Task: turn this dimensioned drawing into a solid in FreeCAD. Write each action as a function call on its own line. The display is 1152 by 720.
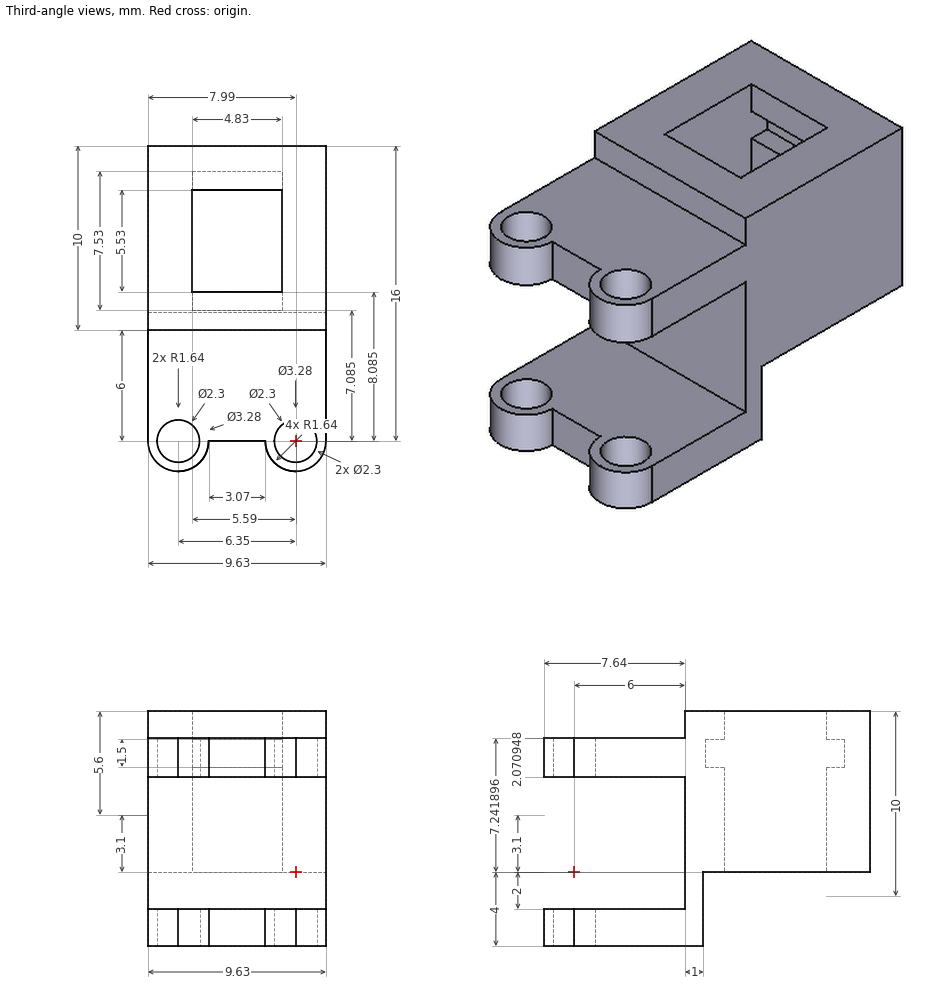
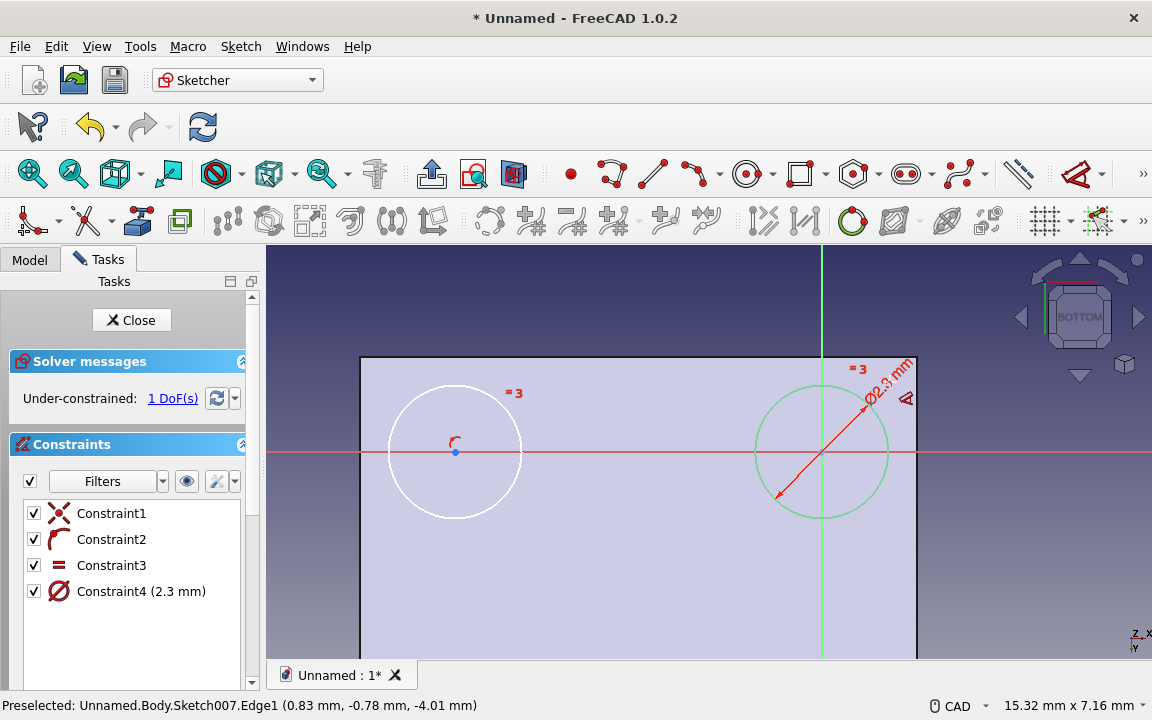
click(455, 452)
click(638, 486)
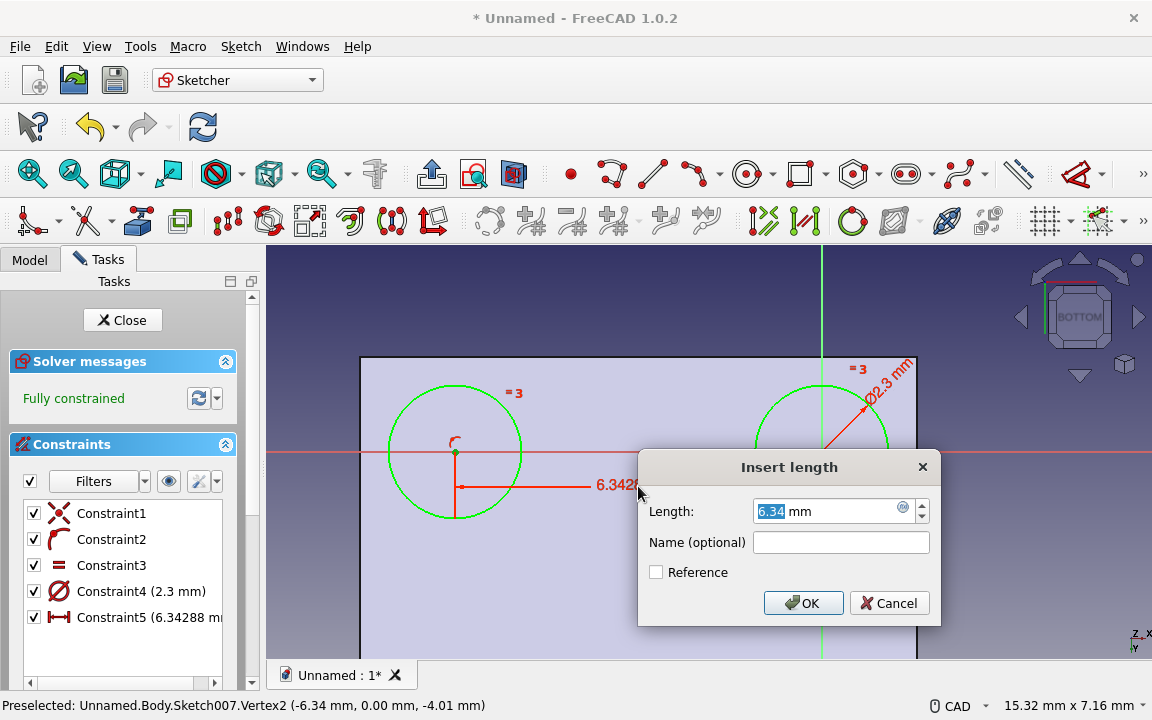
text(6.35)
key(Return)
key(Escape)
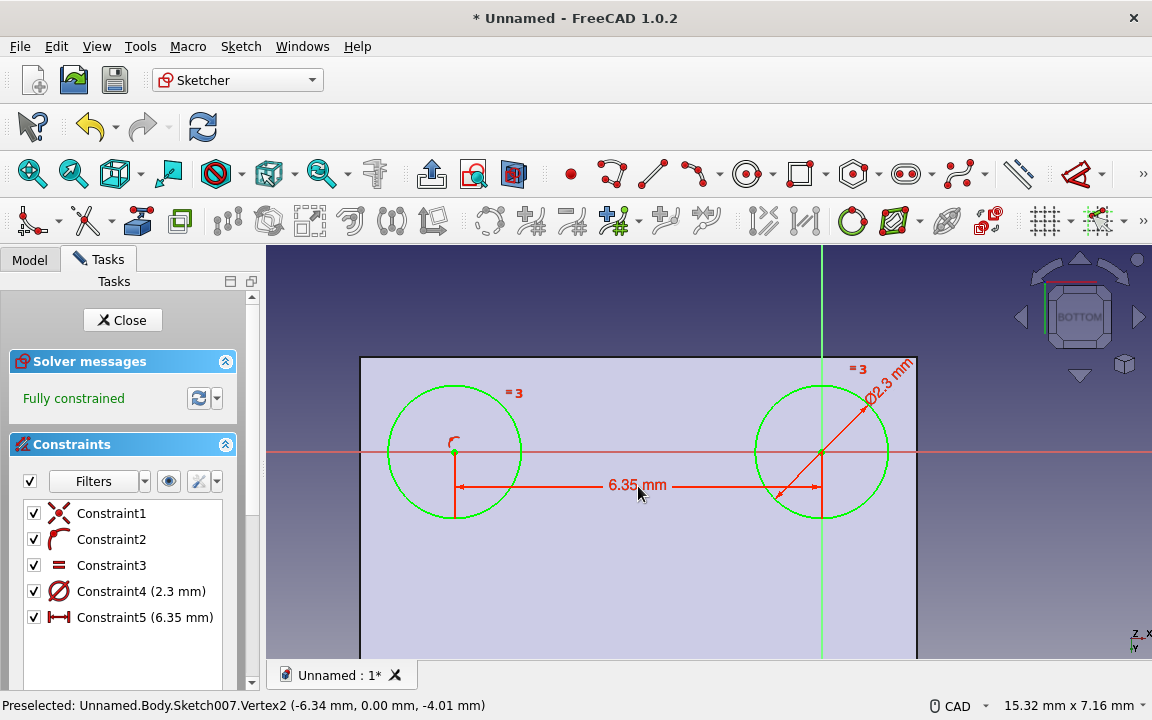
click(123, 320)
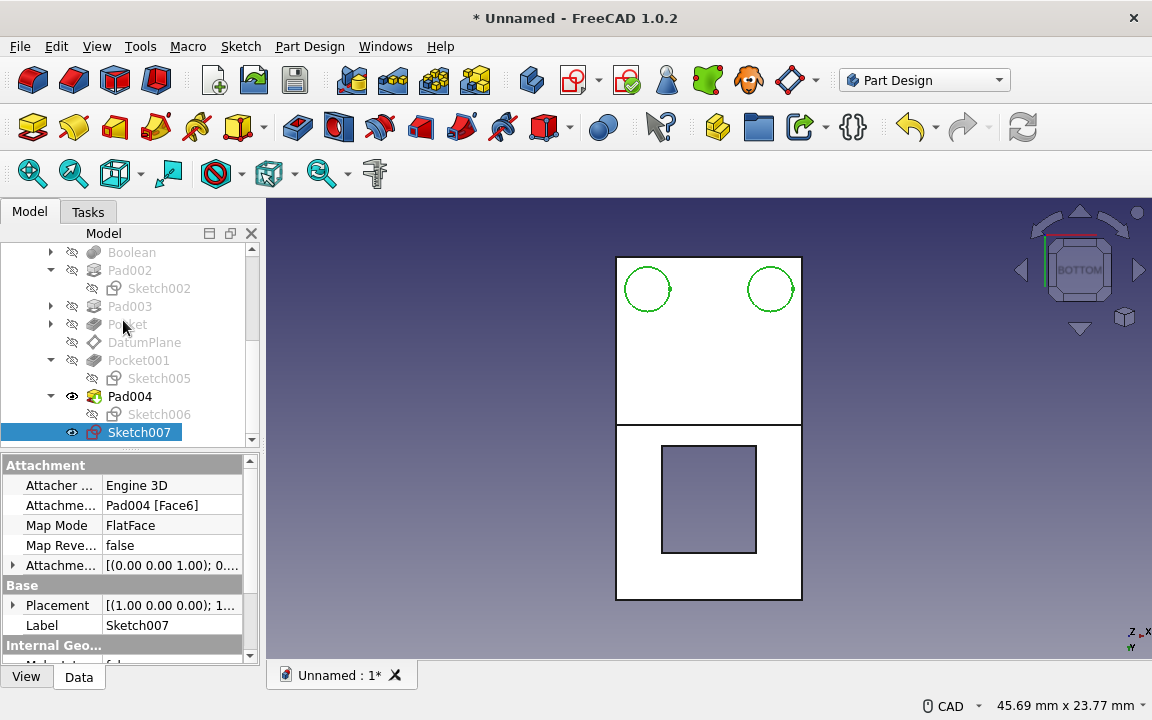
click(298, 128)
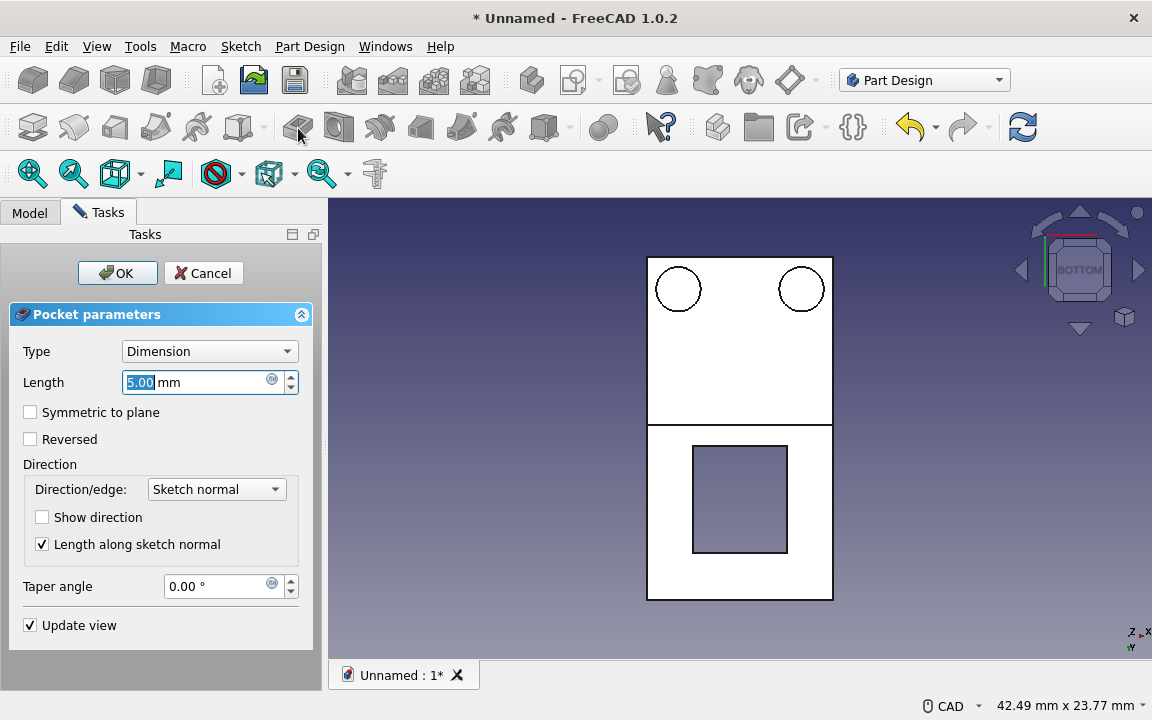
click(210, 352)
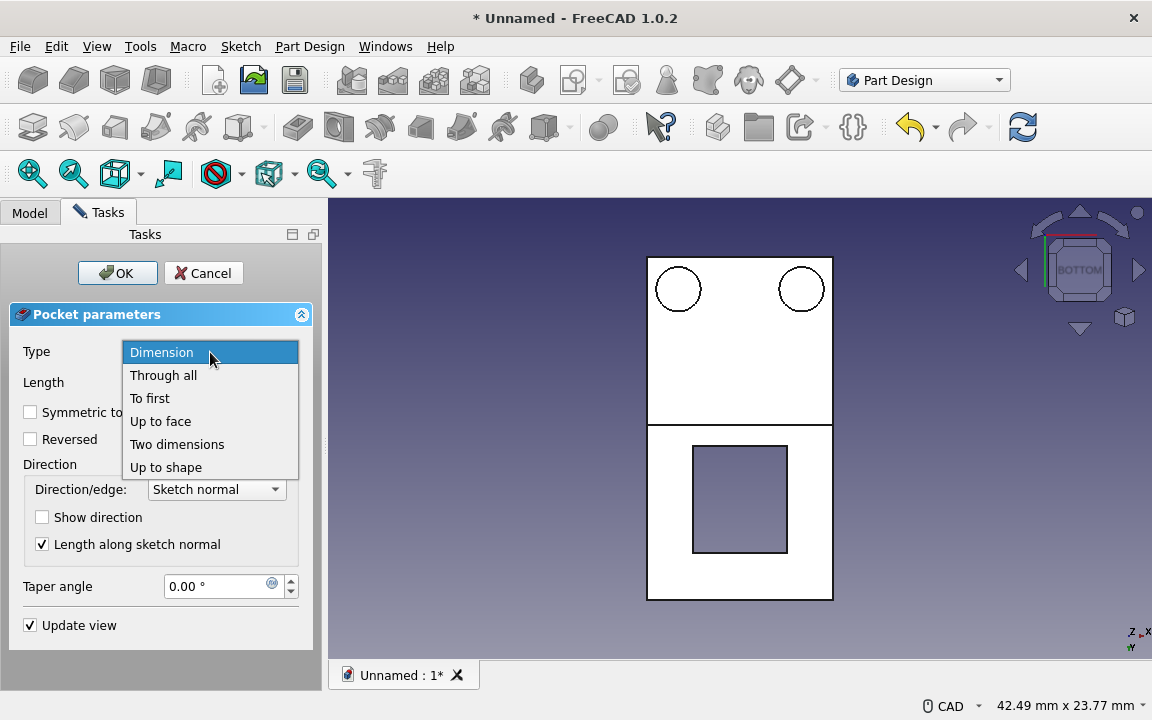
click(208, 376)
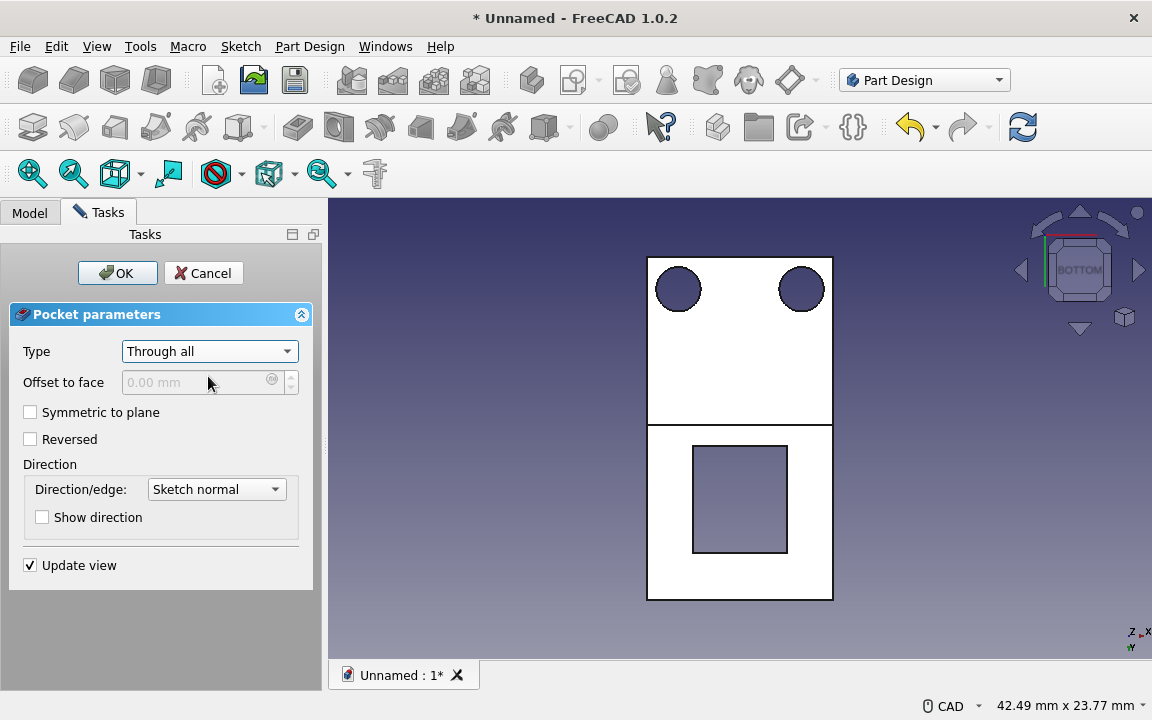
click(118, 273)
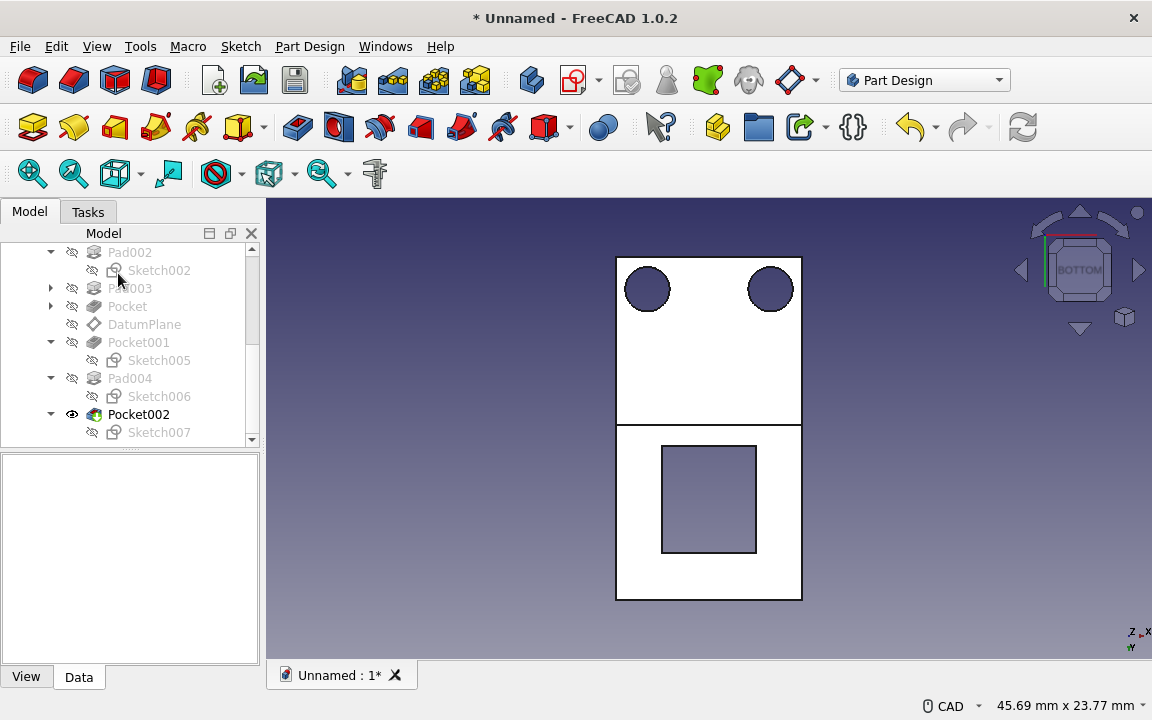
key(0)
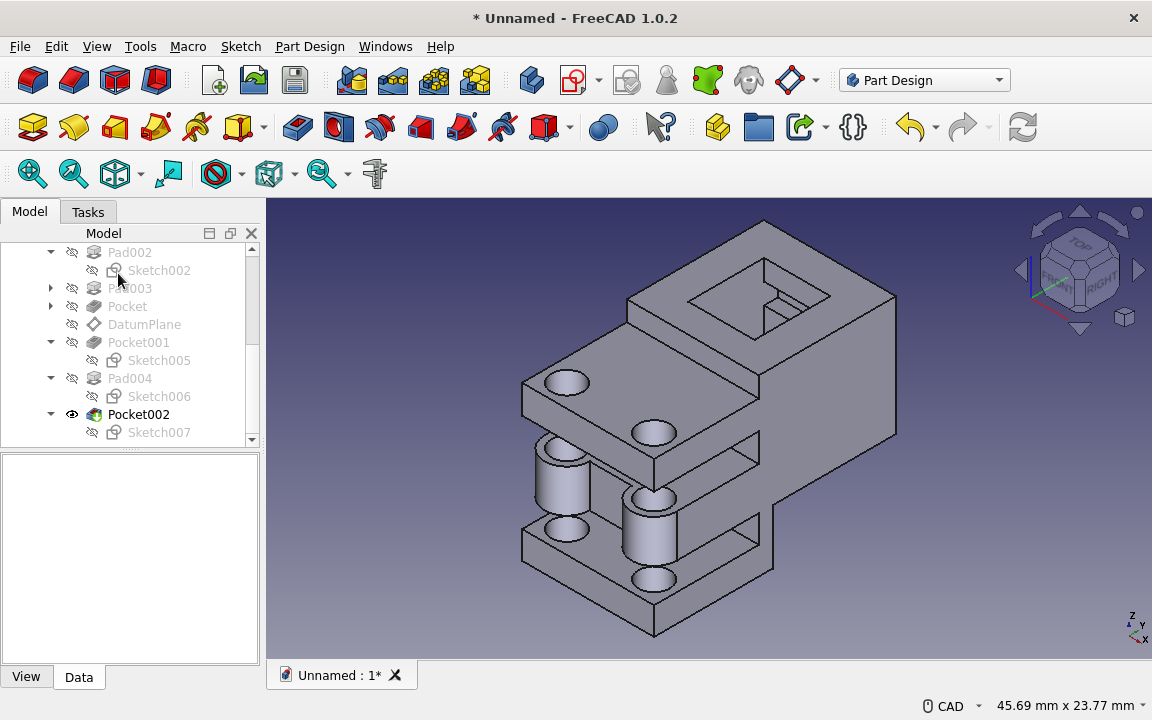
click(844, 397)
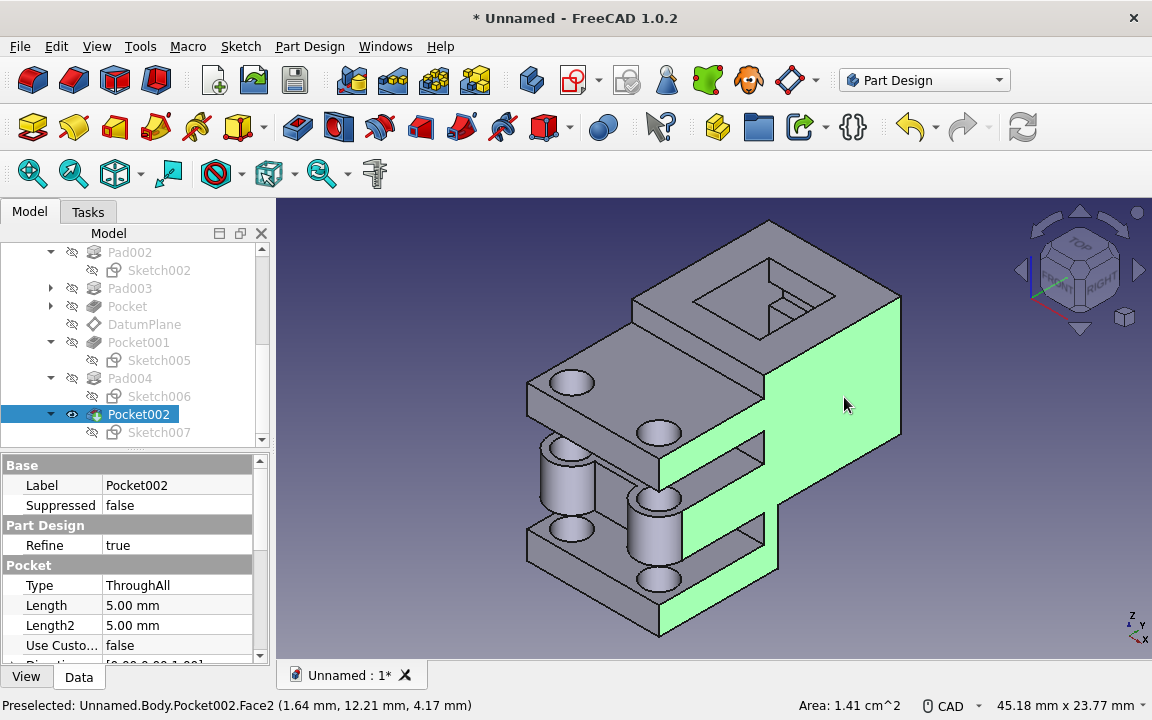
click(572, 80)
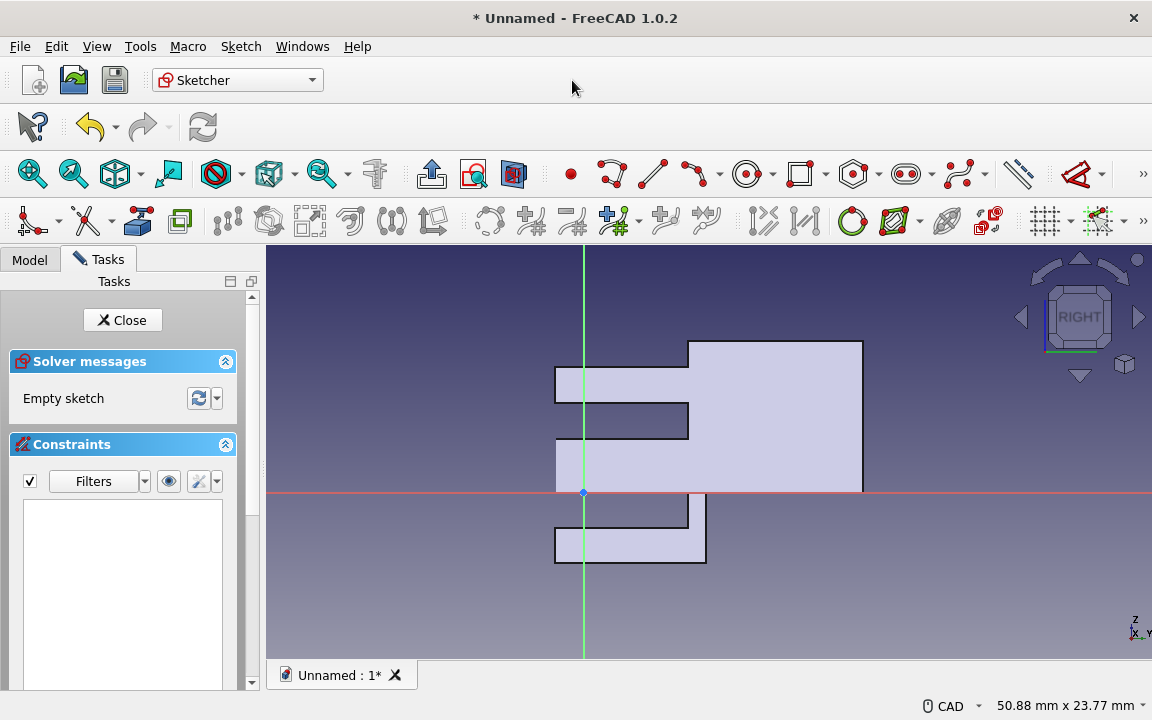
scroll(616, 470, up, 7)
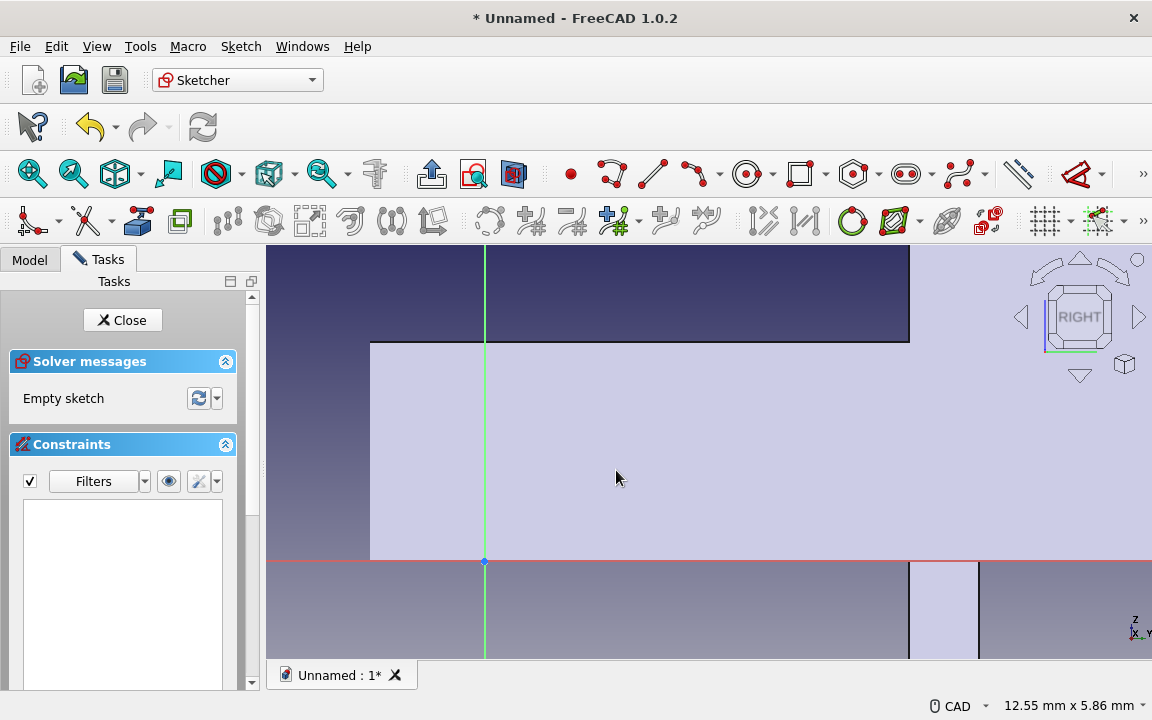
click(800, 174)